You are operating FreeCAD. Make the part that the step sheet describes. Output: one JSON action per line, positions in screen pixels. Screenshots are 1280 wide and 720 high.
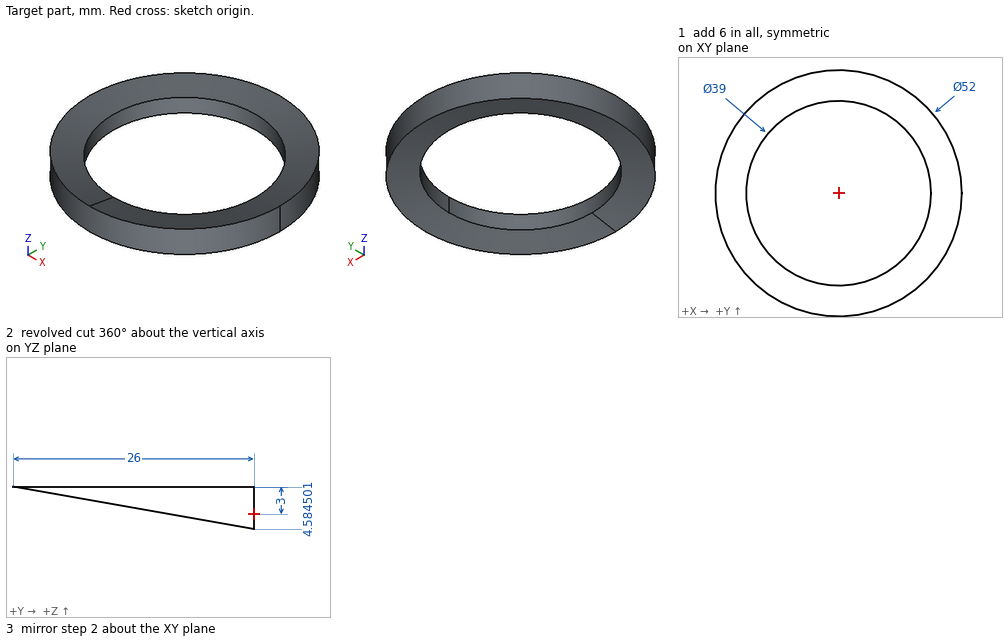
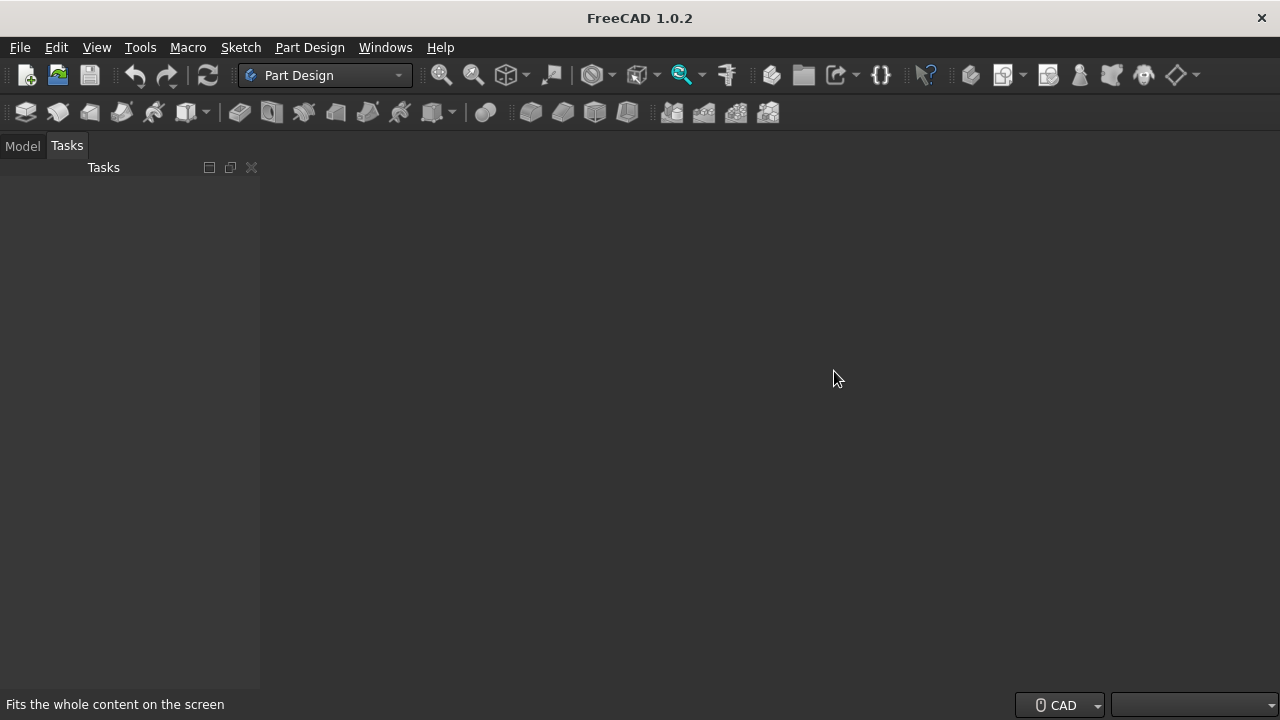
{"action": "key", "text": "ctrl+n"}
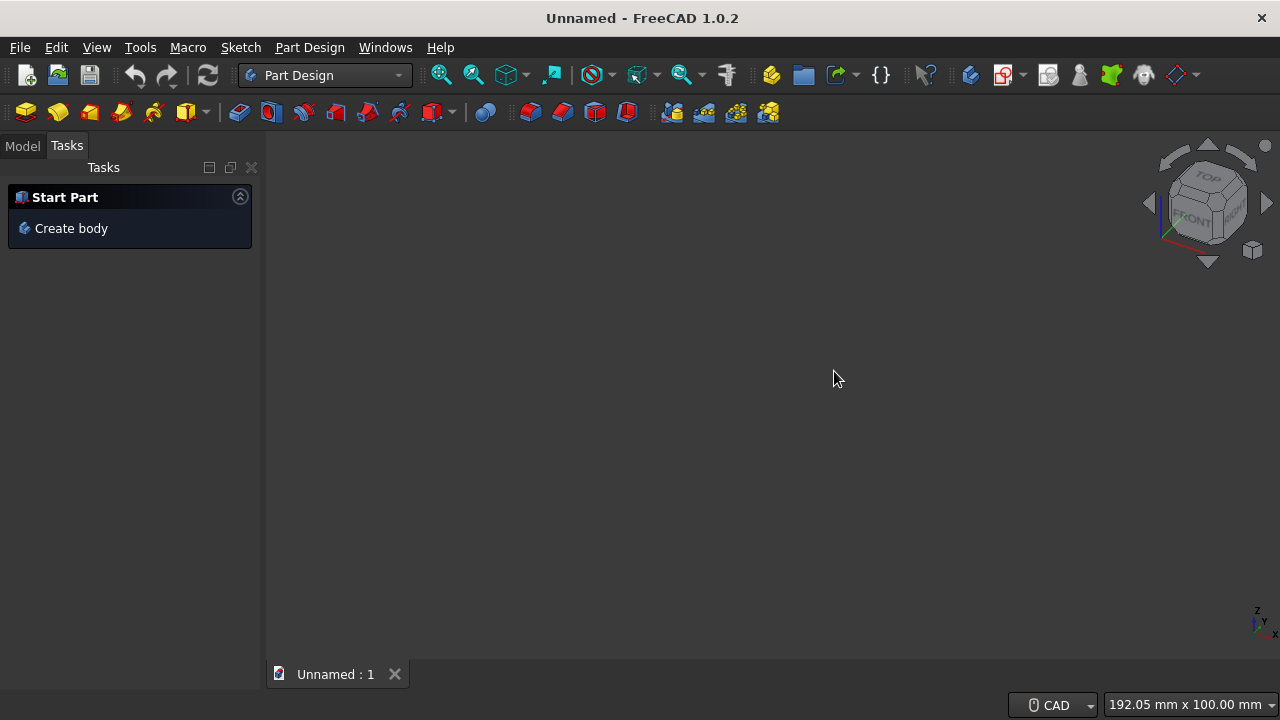
{"action": "left_click", "coordinate": [1004, 76]}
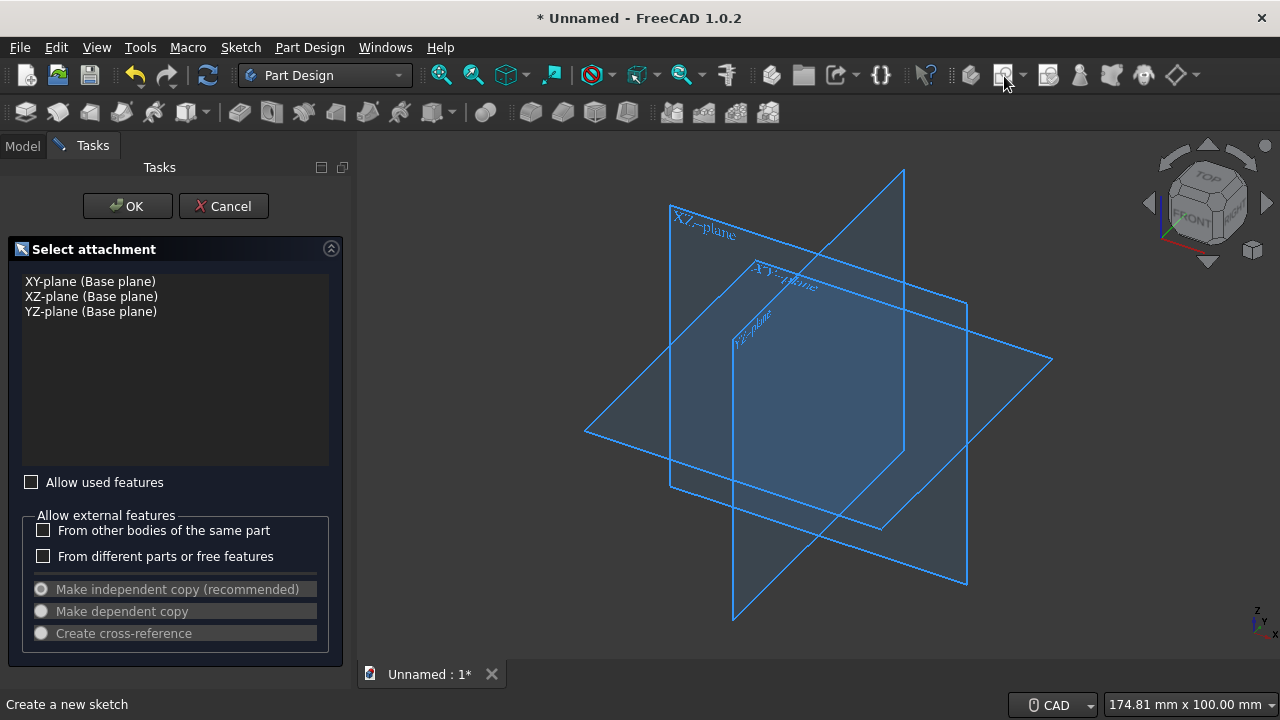
{"action": "left_click", "coordinate": [82, 282]}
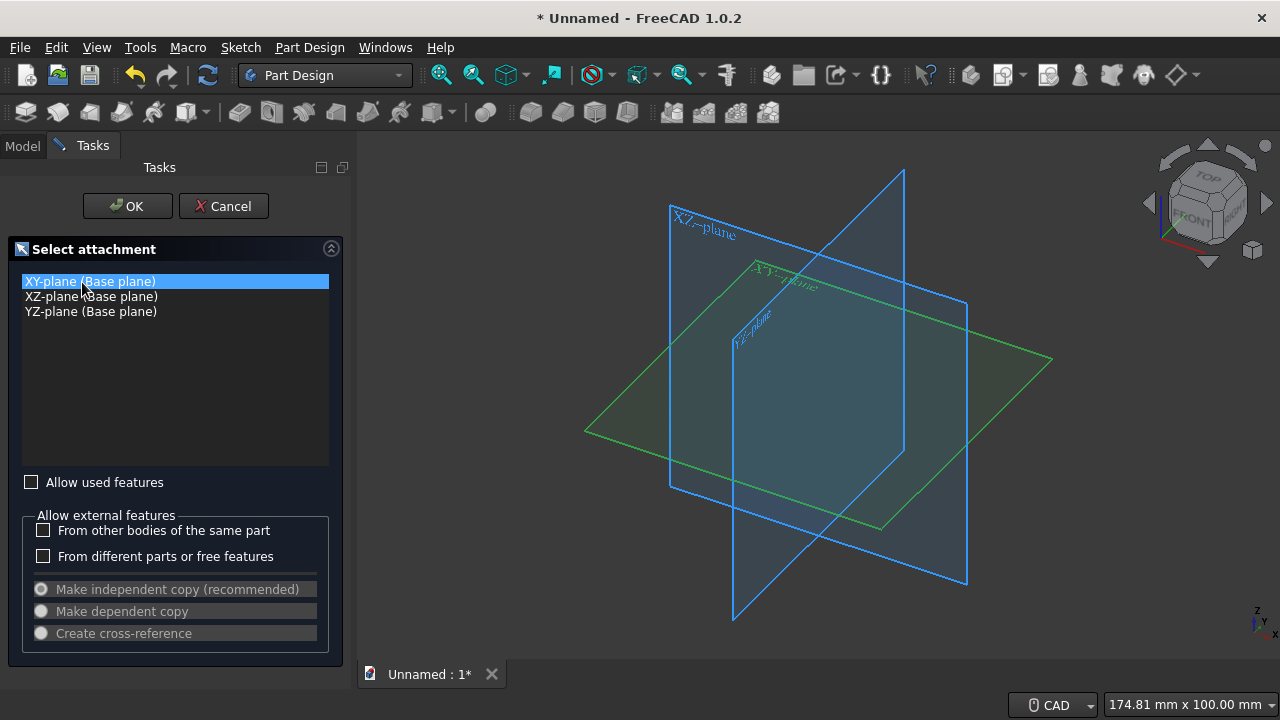
{"action": "left_click", "coordinate": [128, 206]}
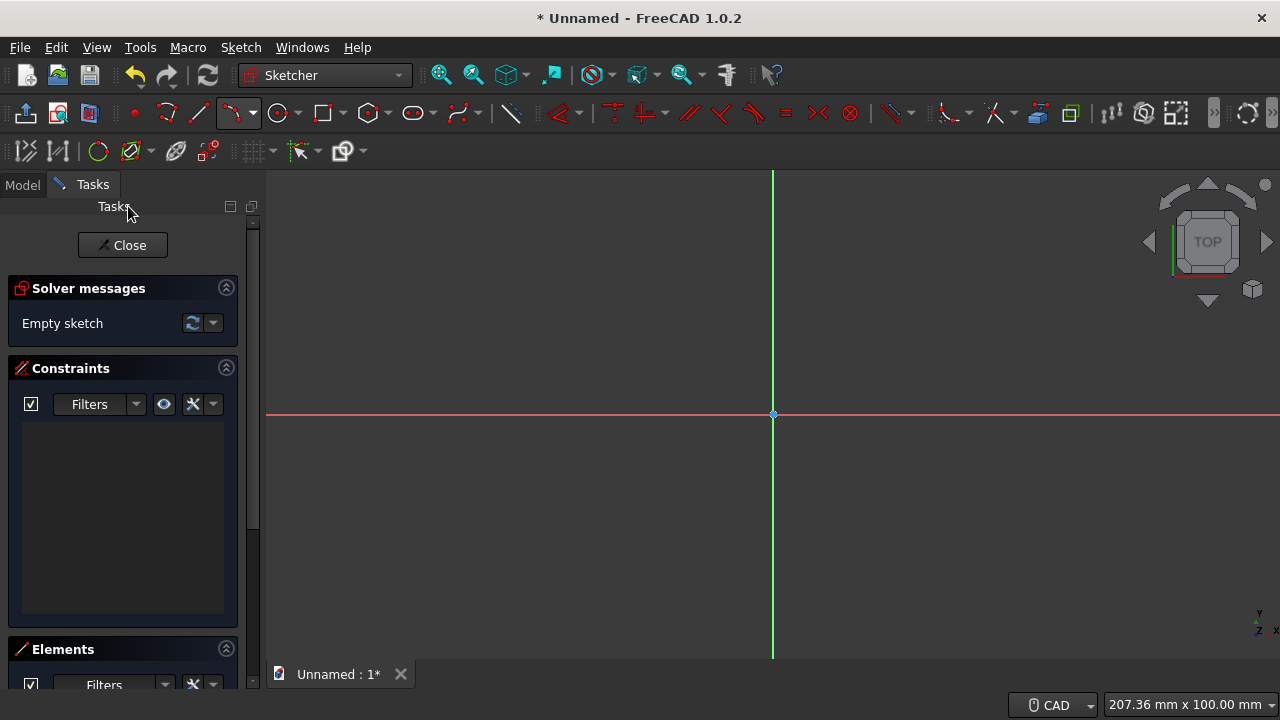
{"action": "left_click", "coordinate": [278, 114]}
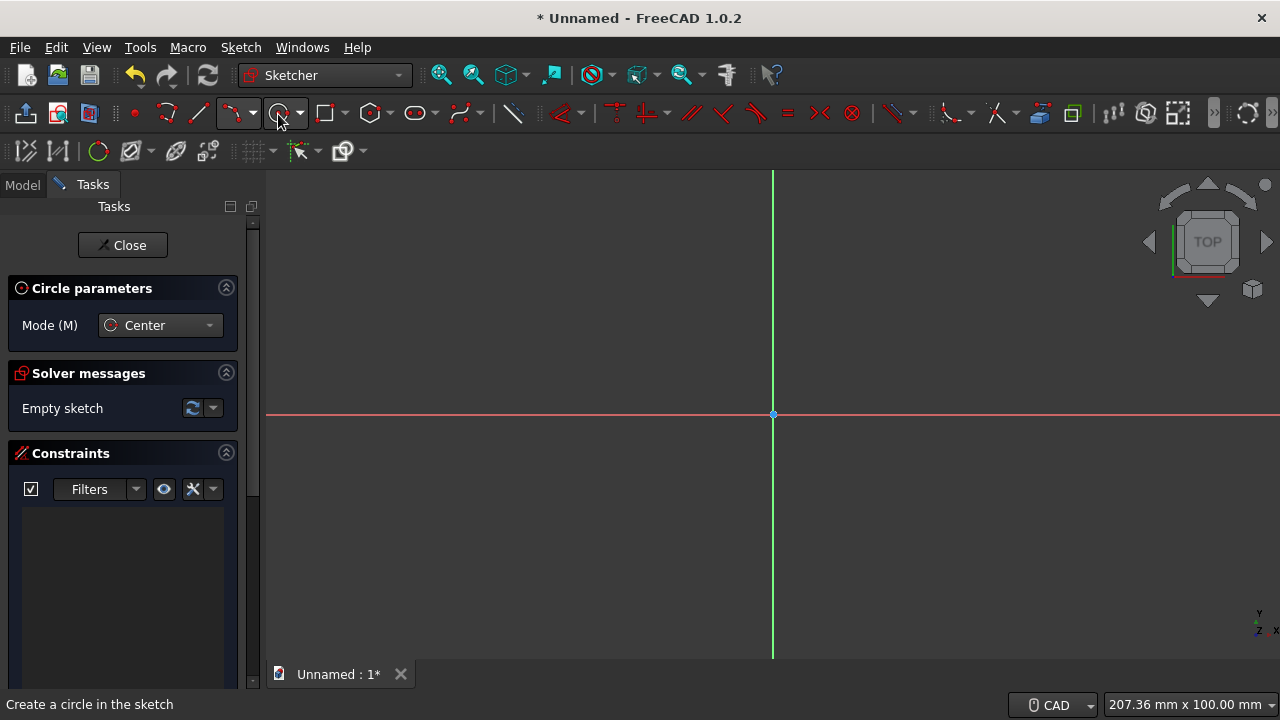
{"action": "left_click", "coordinate": [773, 414]}
{"action": "left_click", "coordinate": [863, 325]}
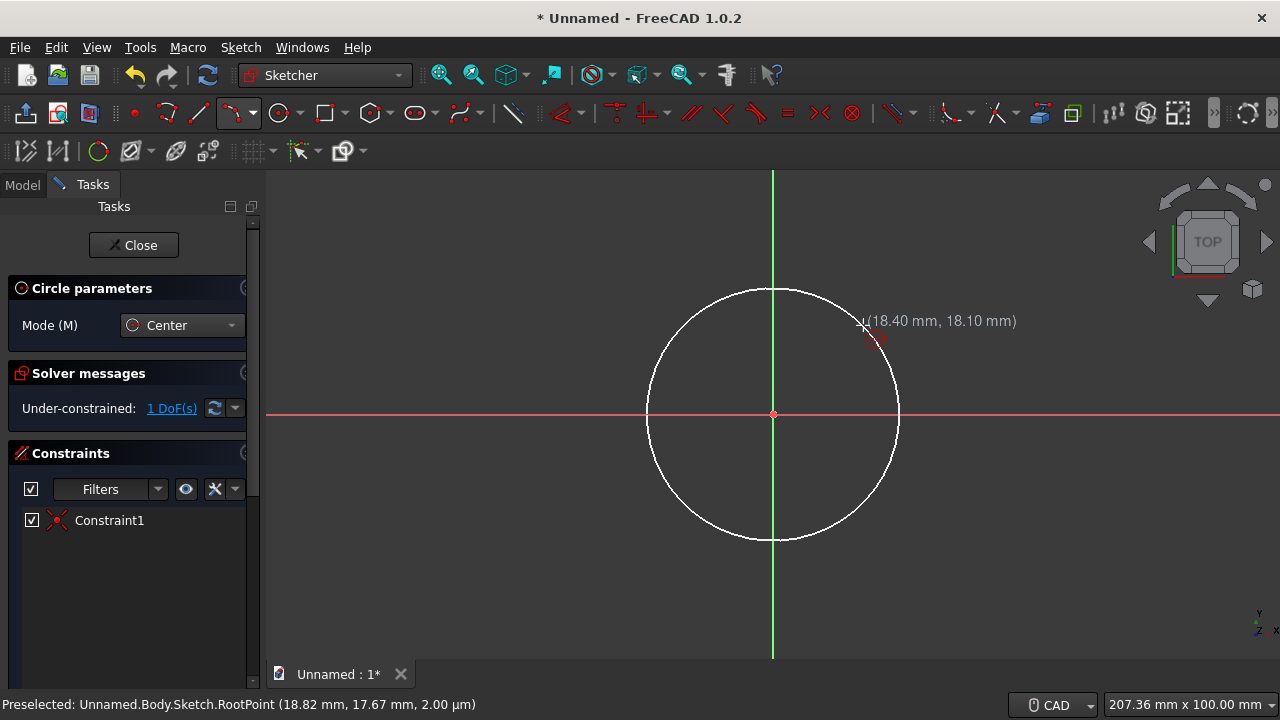
{"action": "left_click", "coordinate": [773, 414]}
{"action": "left_click", "coordinate": [840, 347]}
{"action": "key", "text": "Escape"}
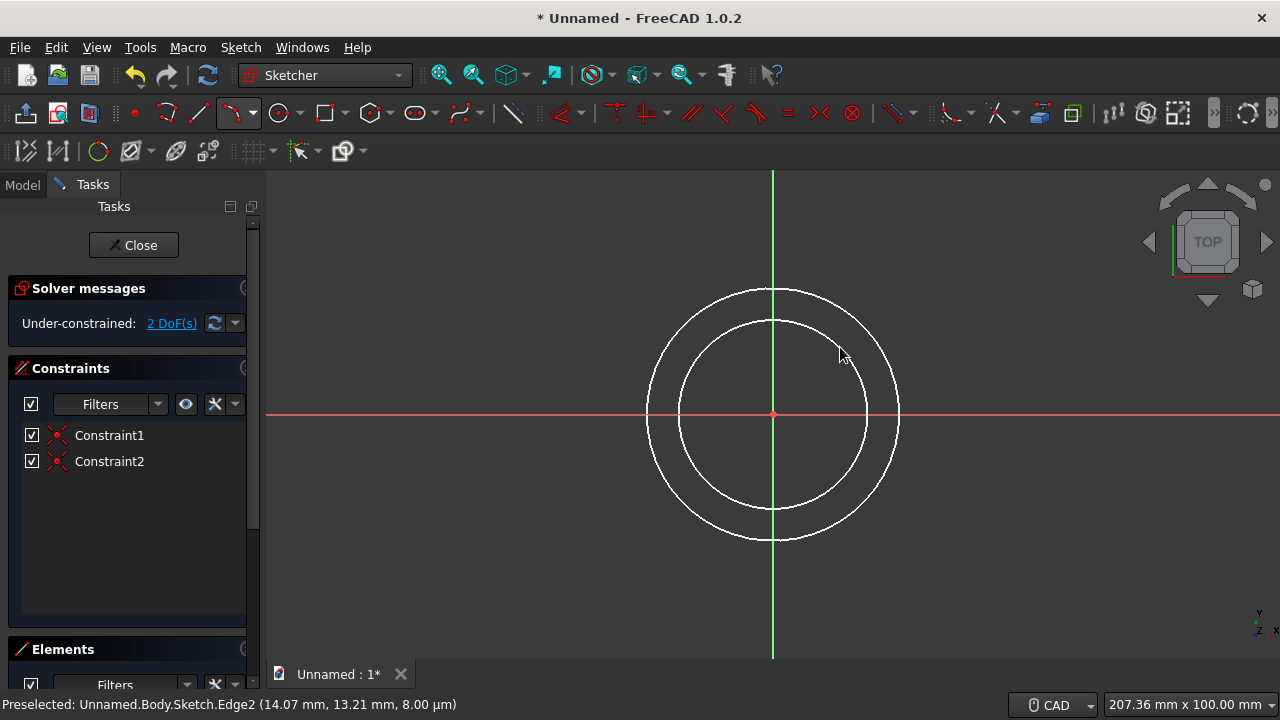
{"action": "left_click", "coordinate": [560, 114]}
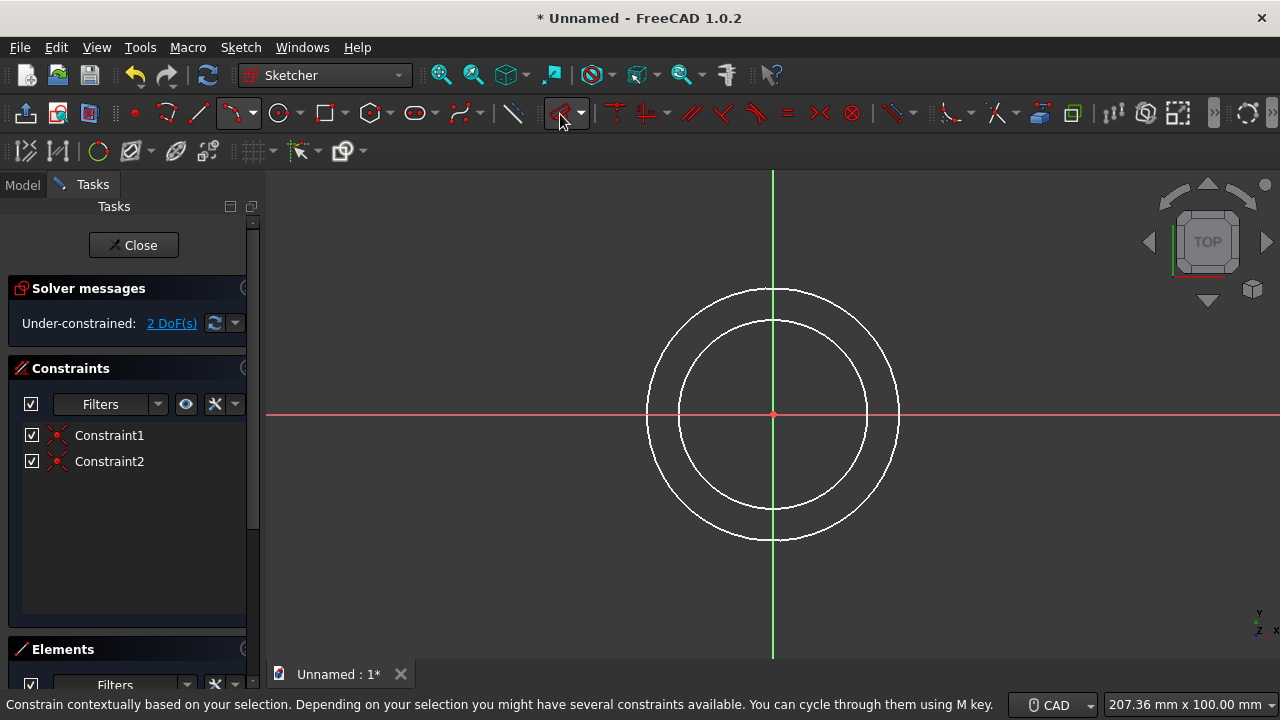
{"action": "left_click", "coordinate": [862, 325]}
{"action": "left_click", "coordinate": [885, 302]}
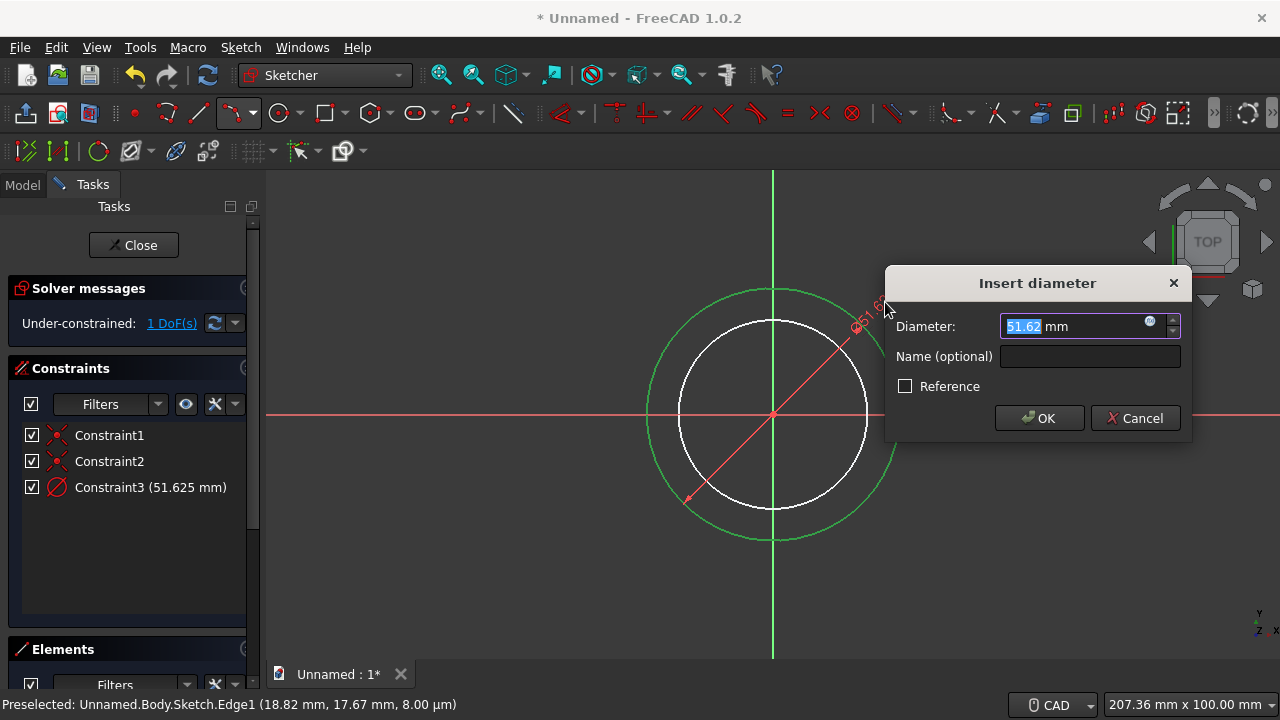
{"action": "type", "text": "52"}
{"action": "key", "text": "Return"}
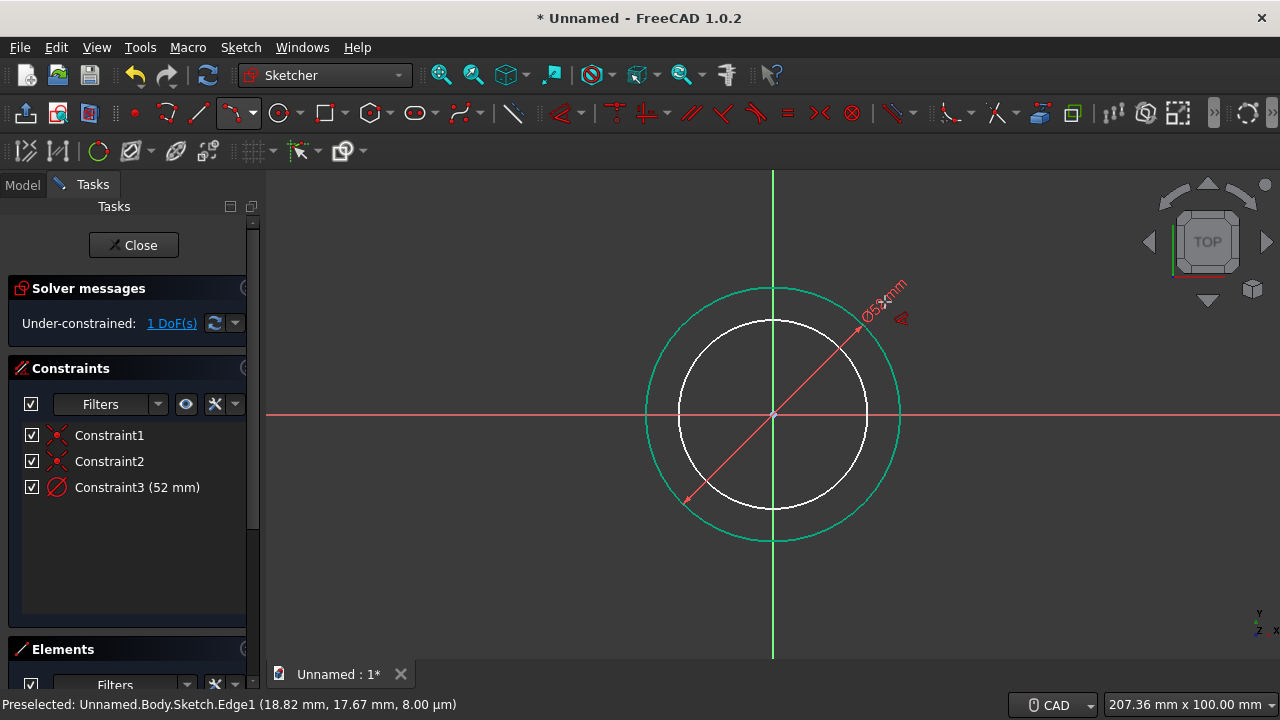
{"action": "left_click", "coordinate": [840, 348]}
{"action": "left_click", "coordinate": [917, 373]}